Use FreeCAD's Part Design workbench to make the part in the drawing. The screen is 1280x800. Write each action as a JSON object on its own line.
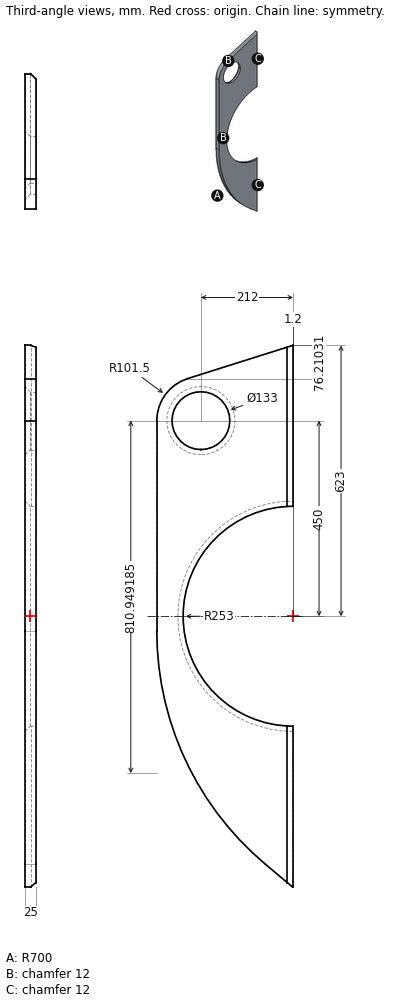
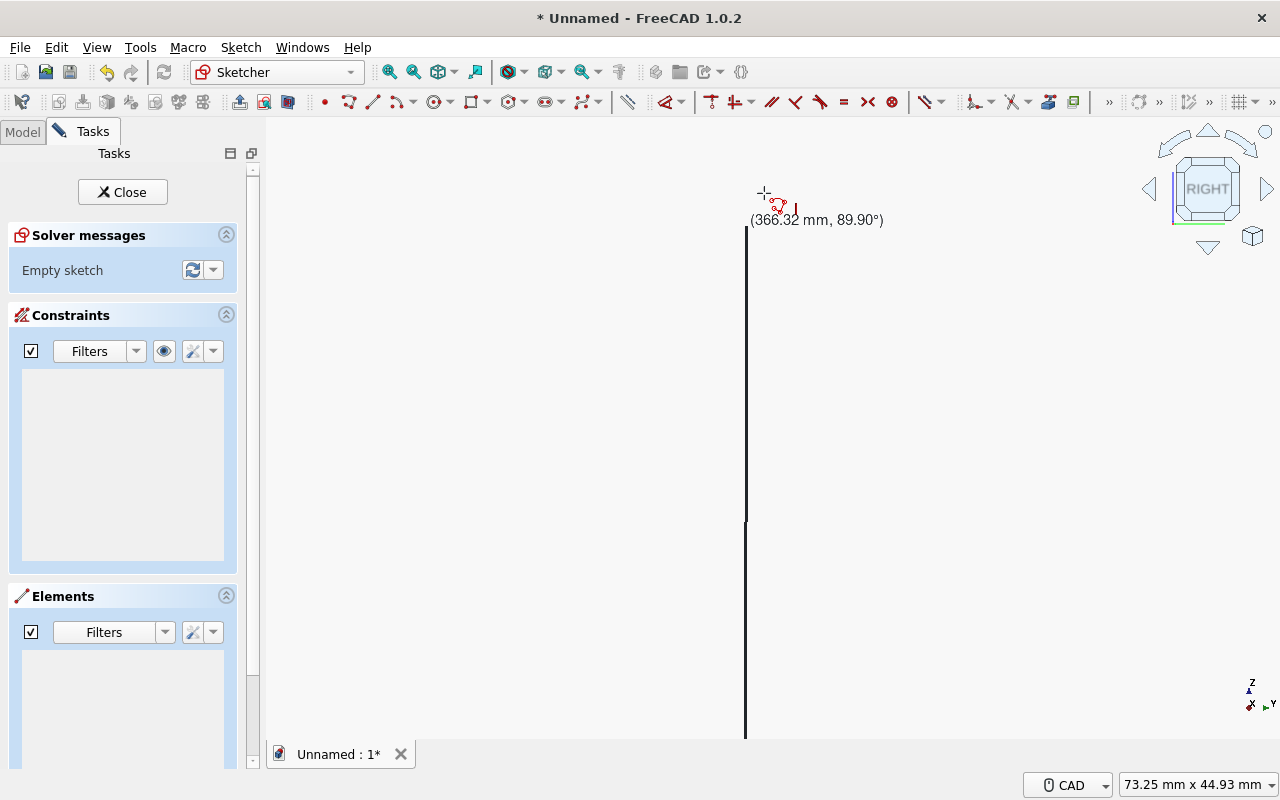
{"action": "left_click", "coordinate": [738, 174]}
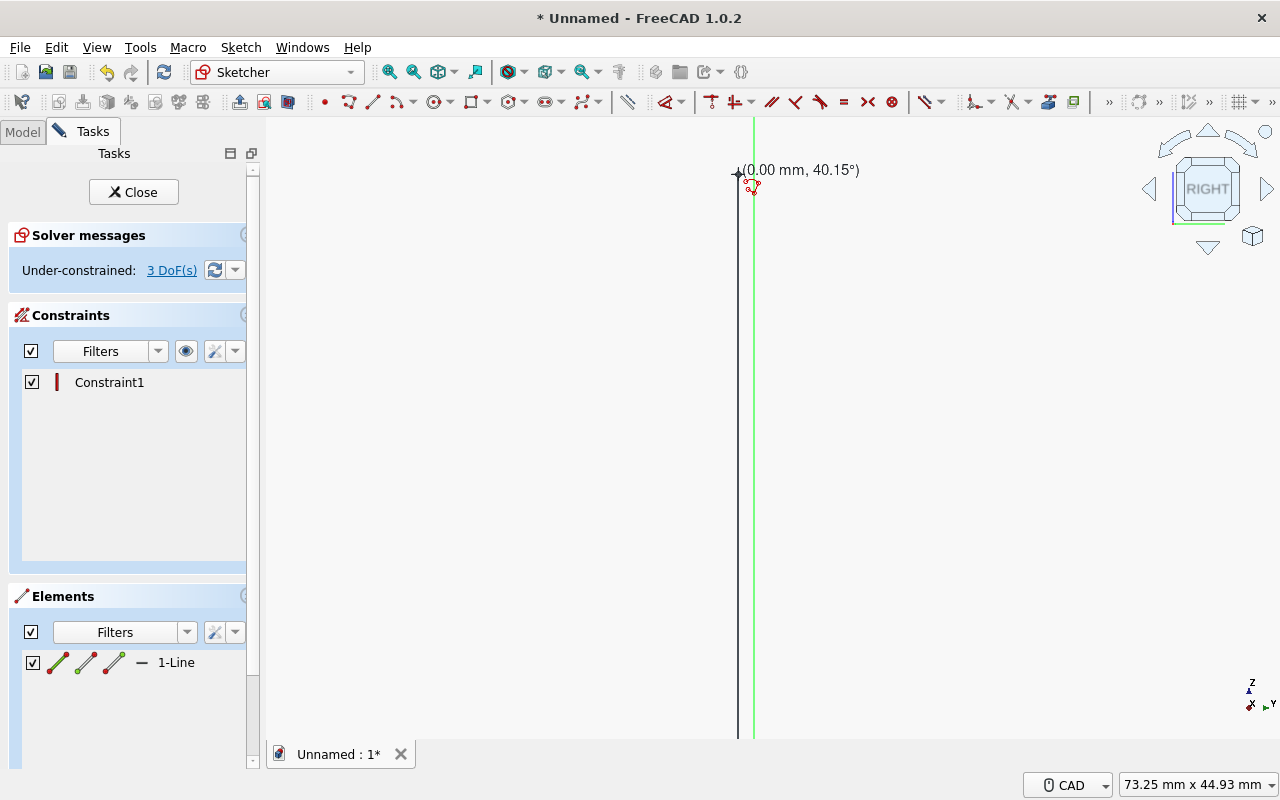
{"action": "scroll", "coordinate": [764, 193], "scroll_direction": "down", "scroll_amount": 18}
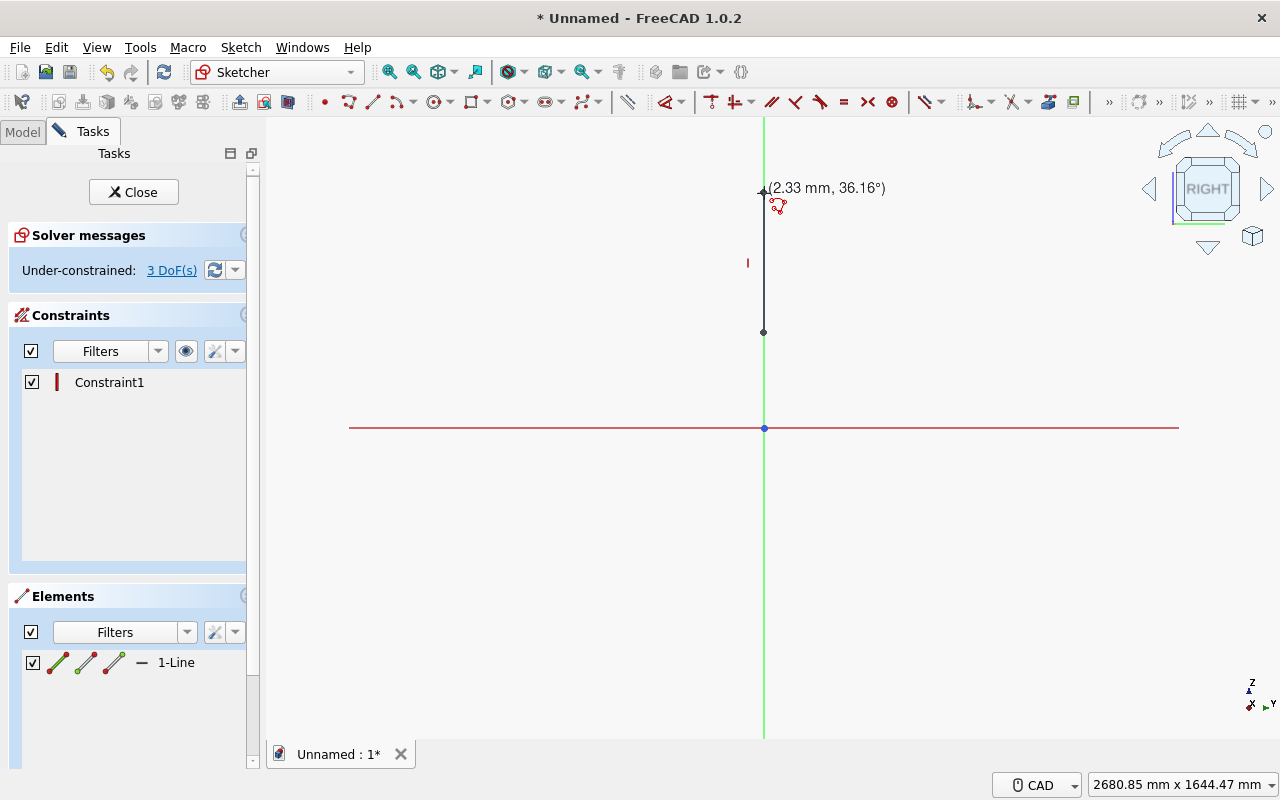
{"action": "left_click", "coordinate": [672, 221]}
{"action": "right_click", "coordinate": [672, 221]}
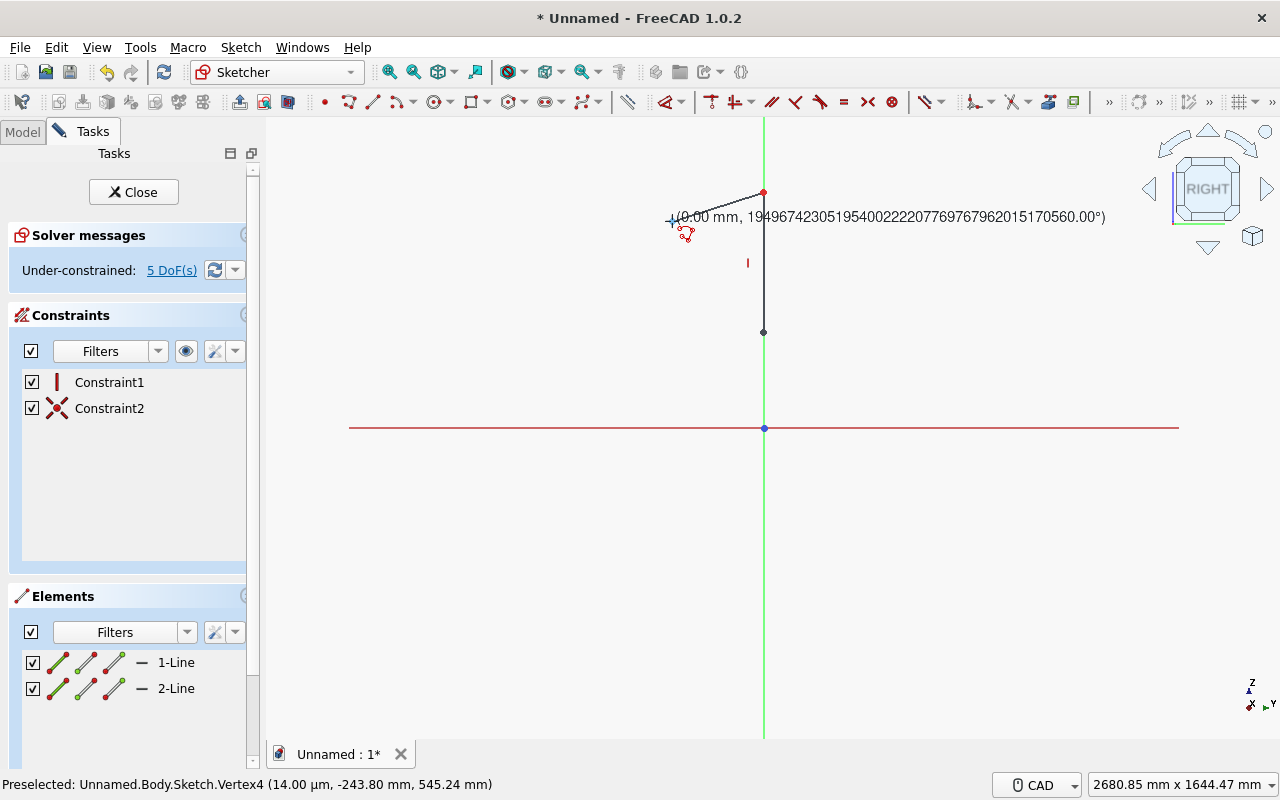
{"action": "left_click", "coordinate": [646, 258]}
{"action": "left_click", "coordinate": [646, 565]}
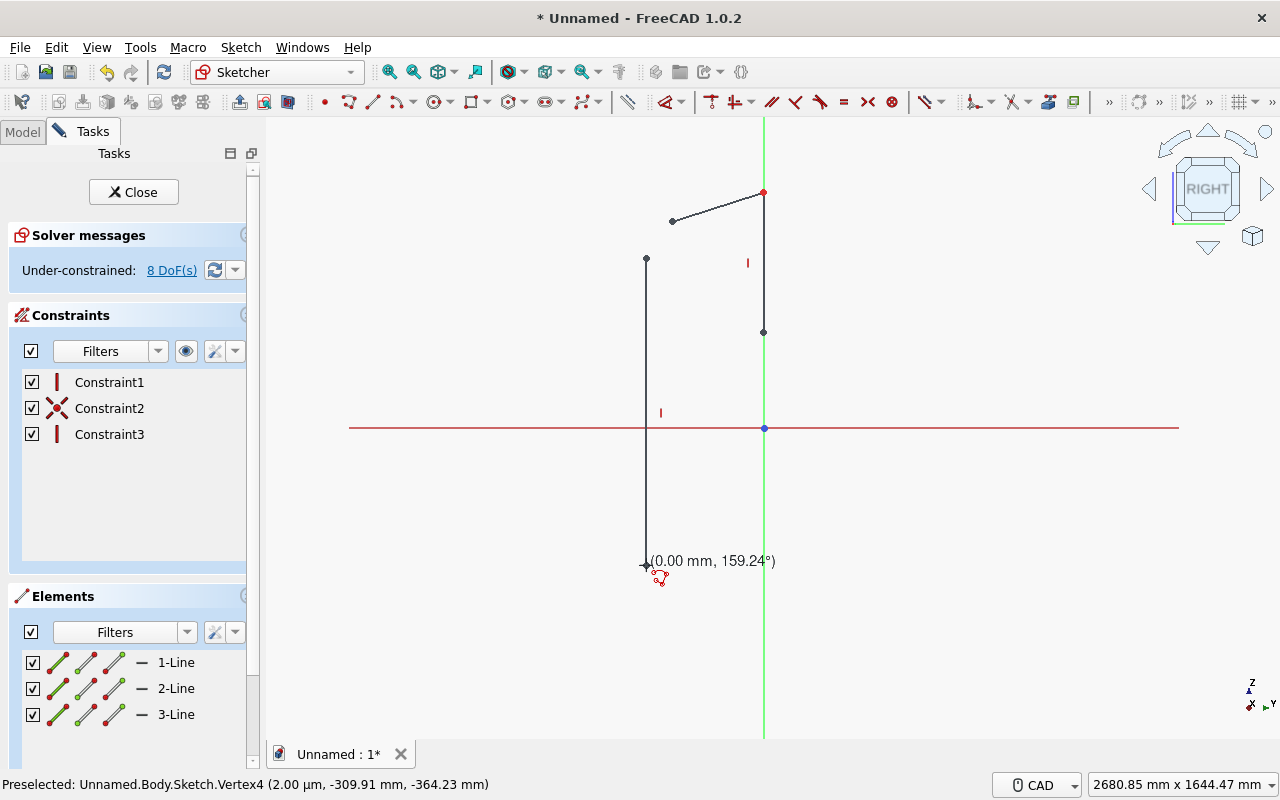
{"action": "scroll", "coordinate": [764, 664], "scroll_direction": "up", "scroll_amount": 18}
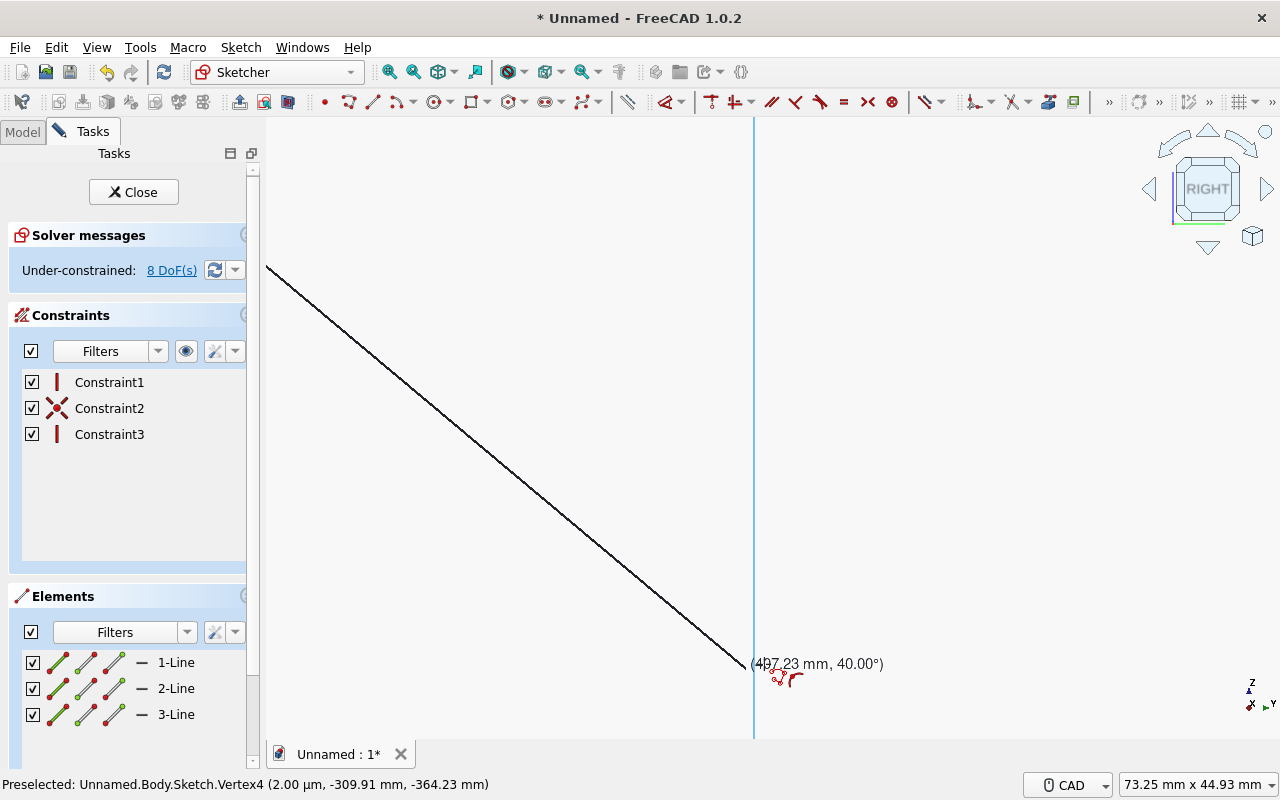
{"action": "left_click", "coordinate": [738, 628]}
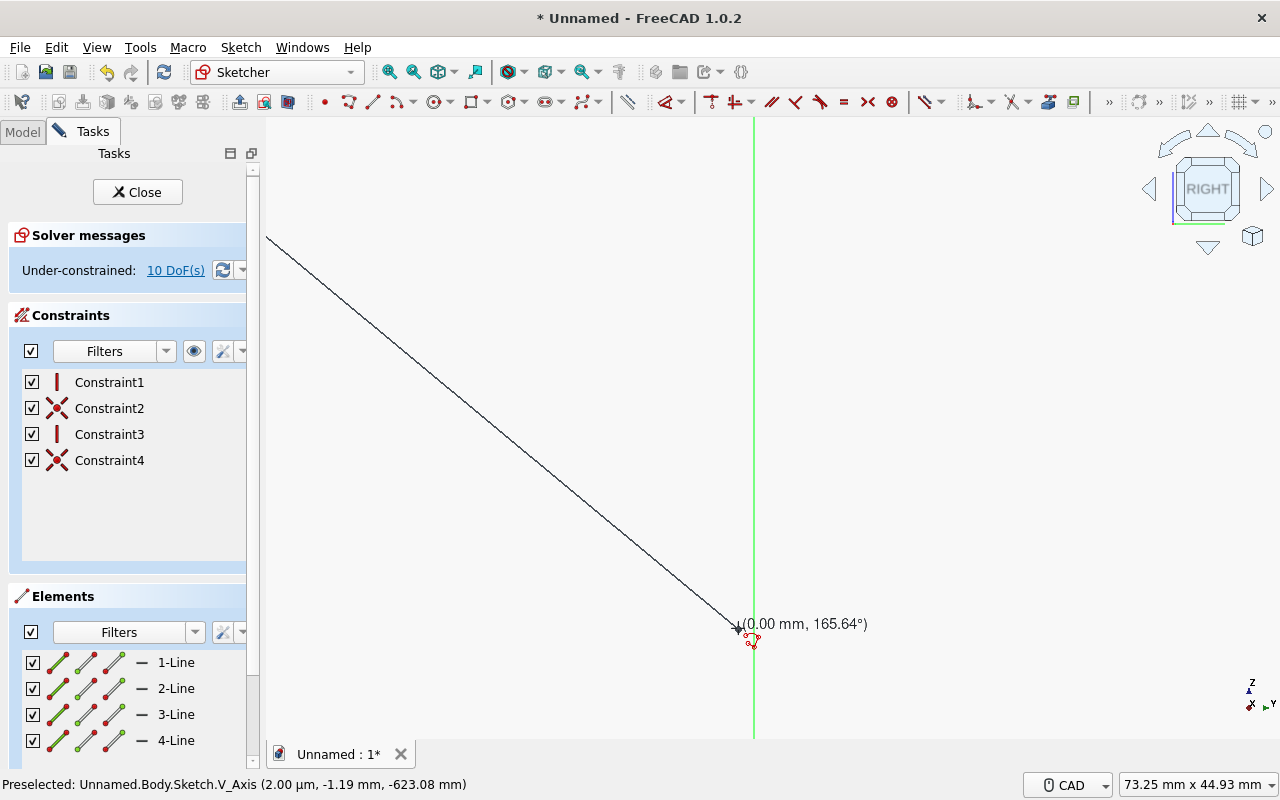
{"action": "scroll", "coordinate": [764, 665], "scroll_direction": "down", "scroll_amount": 18}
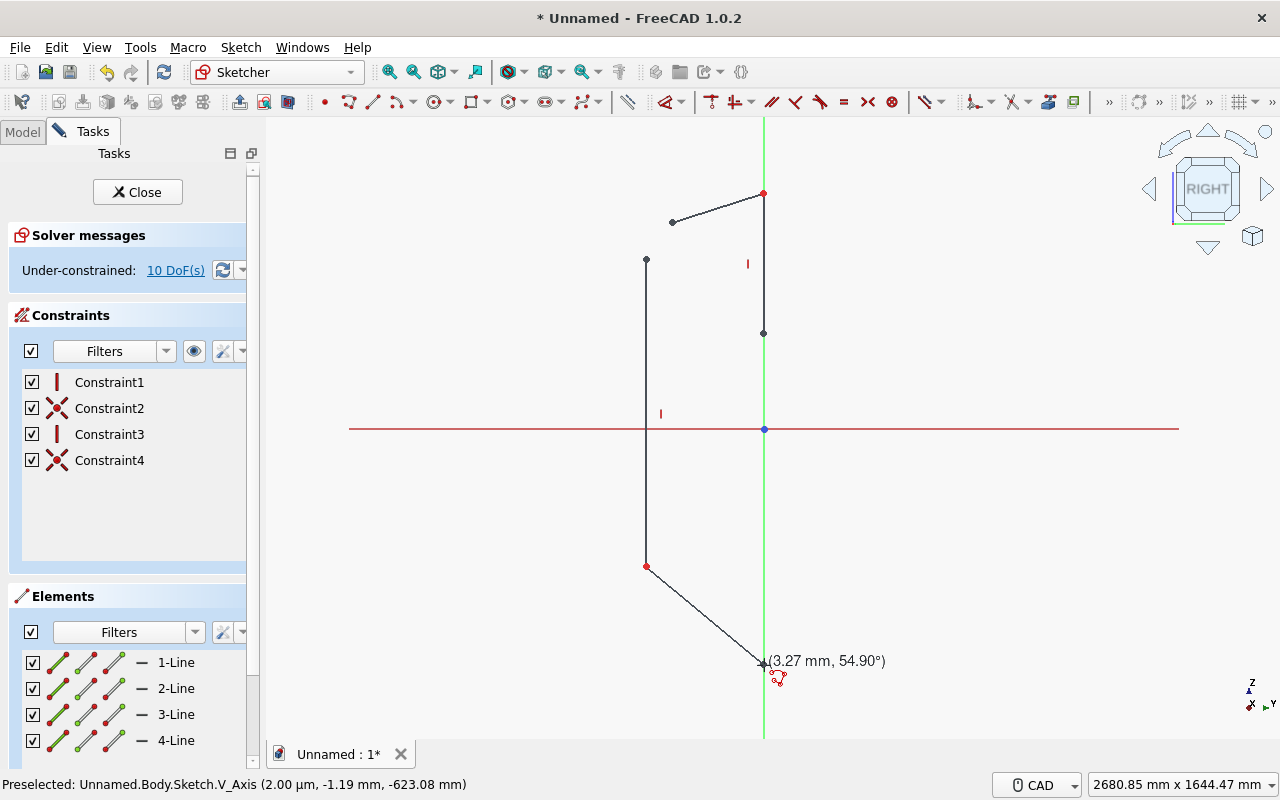
{"action": "scroll", "coordinate": [764, 525], "scroll_direction": "up", "scroll_amount": 18}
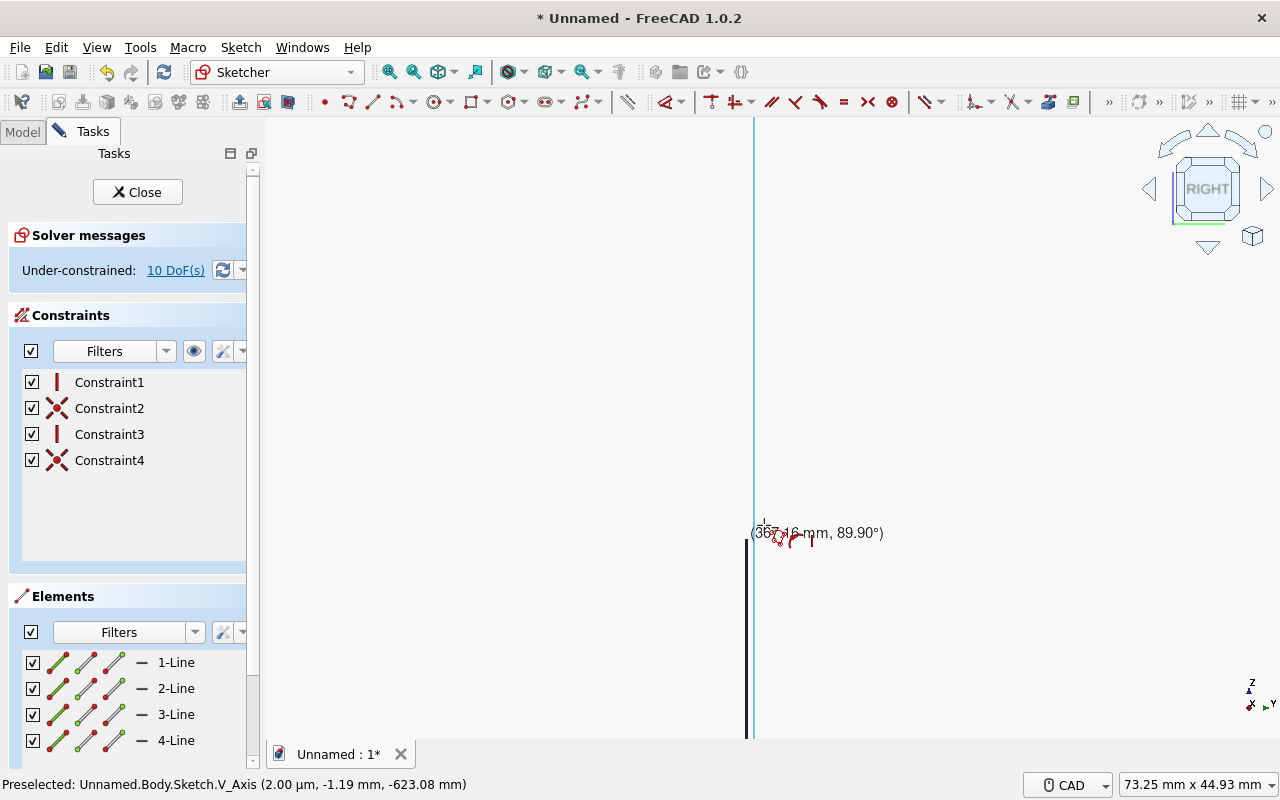
{"action": "left_click", "coordinate": [738, 498]}
{"action": "right_click", "coordinate": [738, 498]}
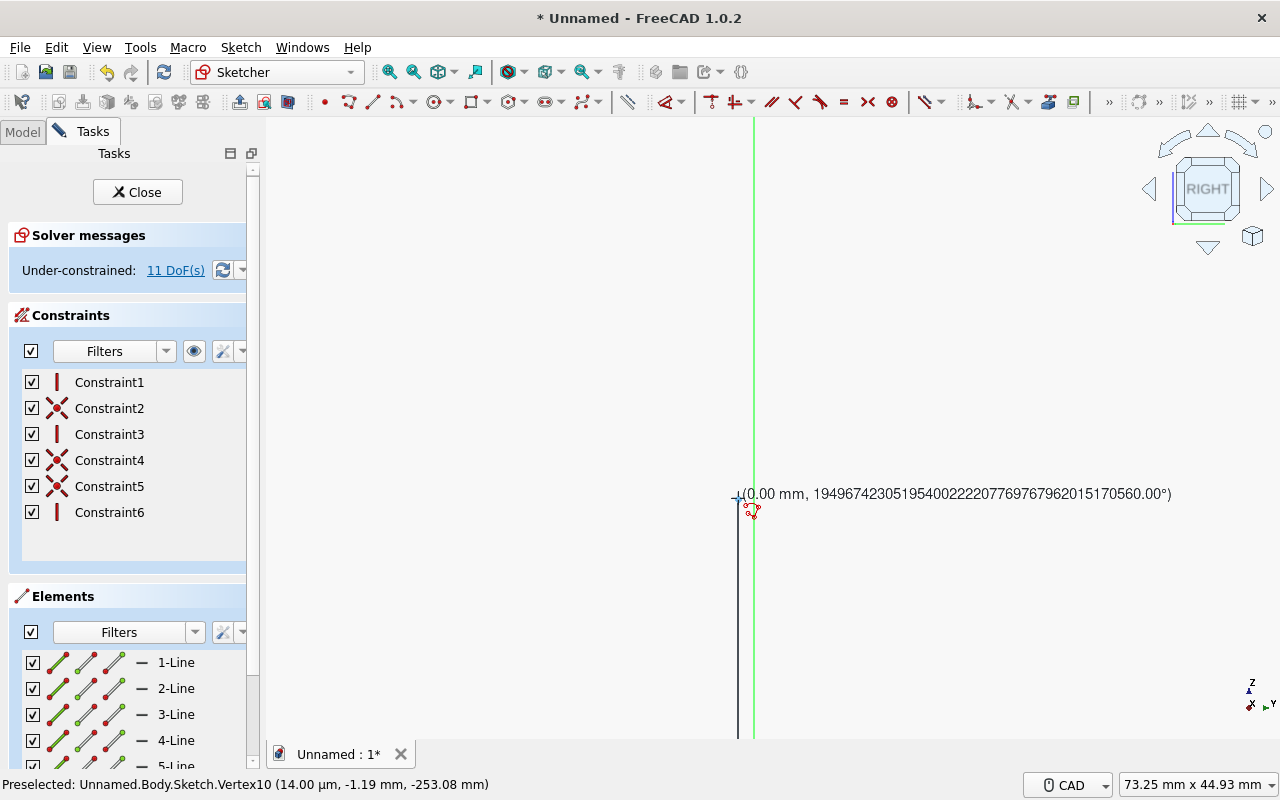
{"action": "left_click", "coordinate": [416, 102]}